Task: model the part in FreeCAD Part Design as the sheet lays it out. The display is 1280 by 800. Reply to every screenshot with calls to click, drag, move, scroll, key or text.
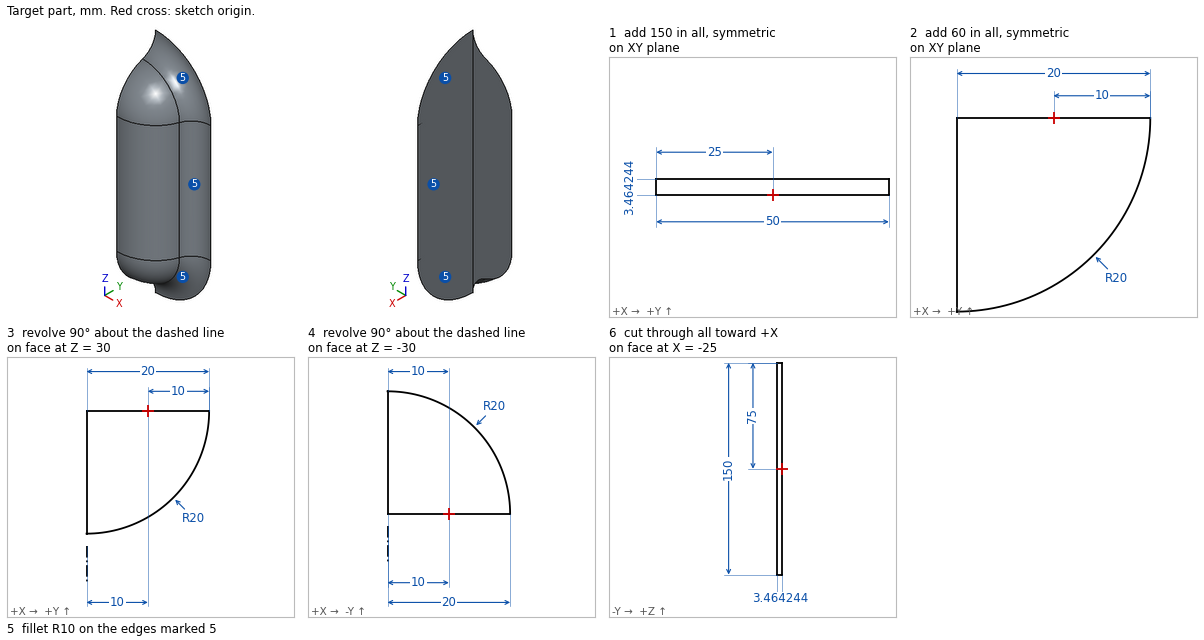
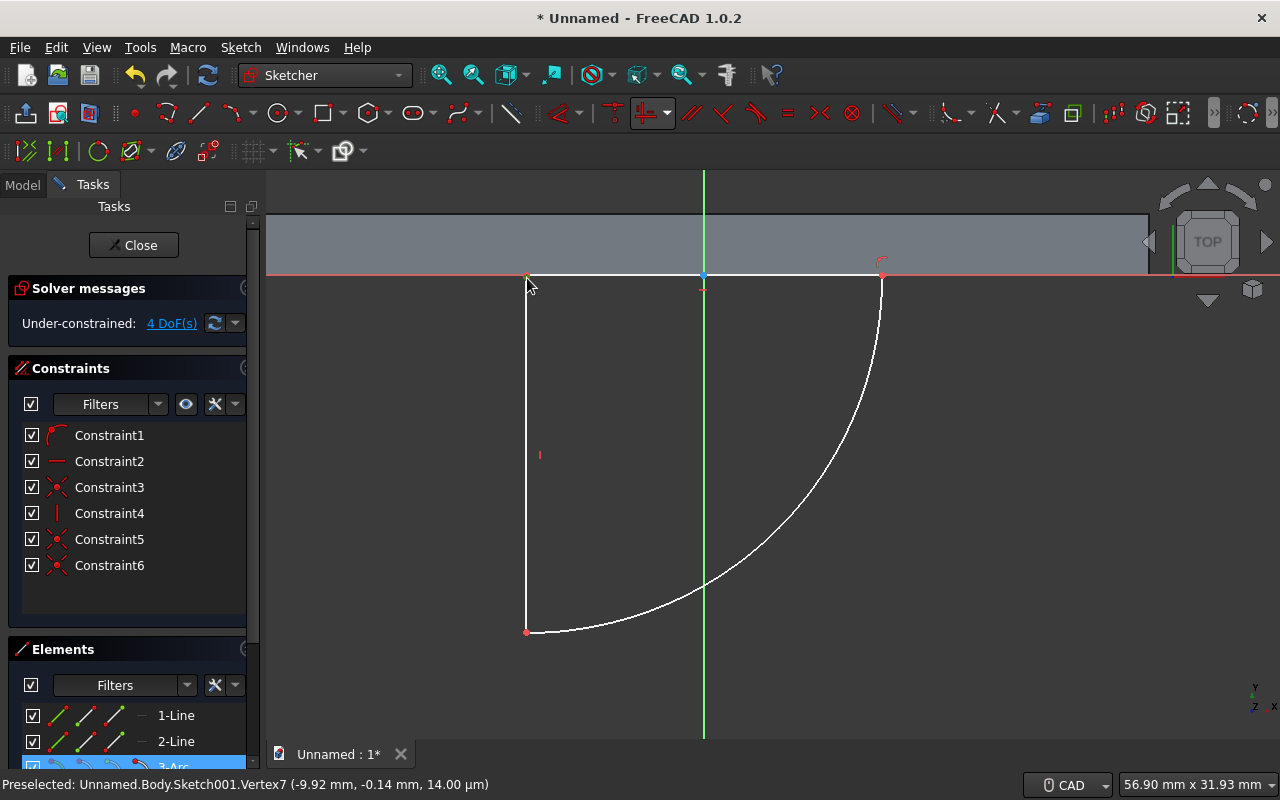
click(353, 275)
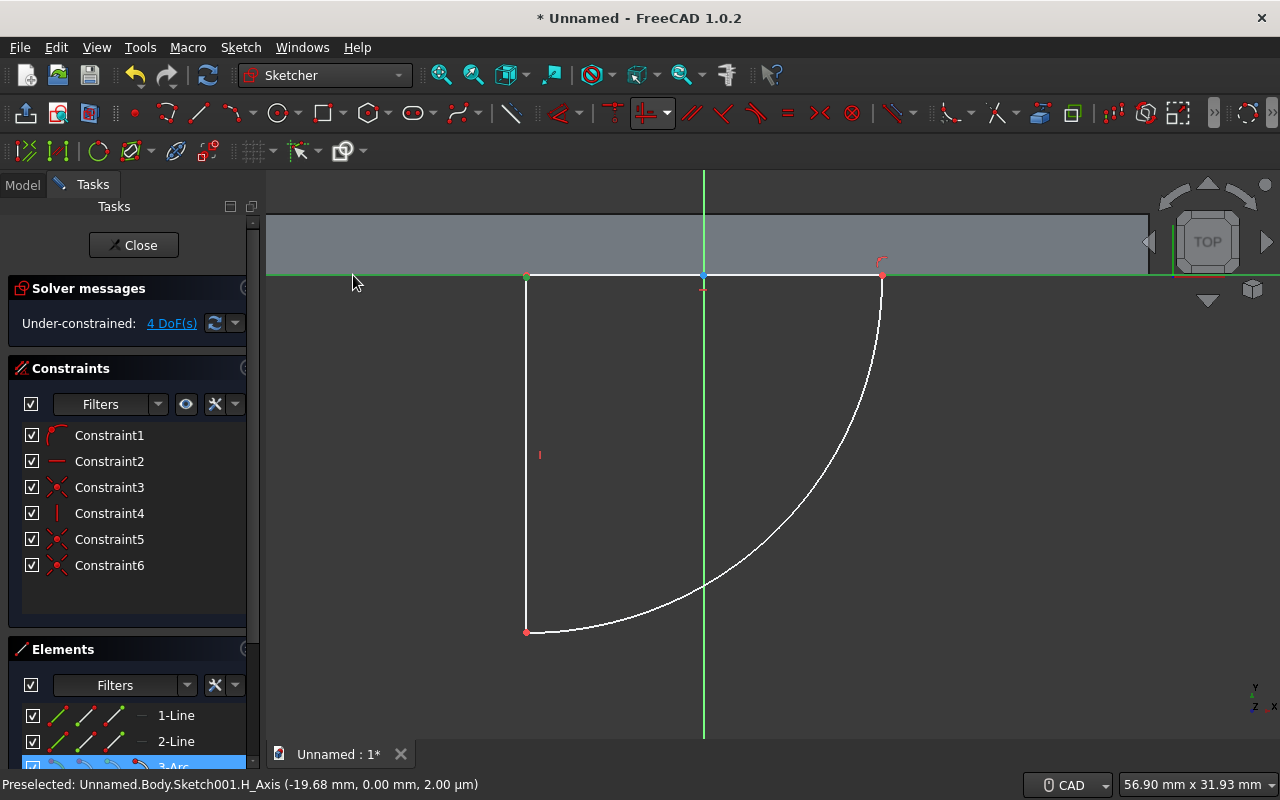
click(614, 114)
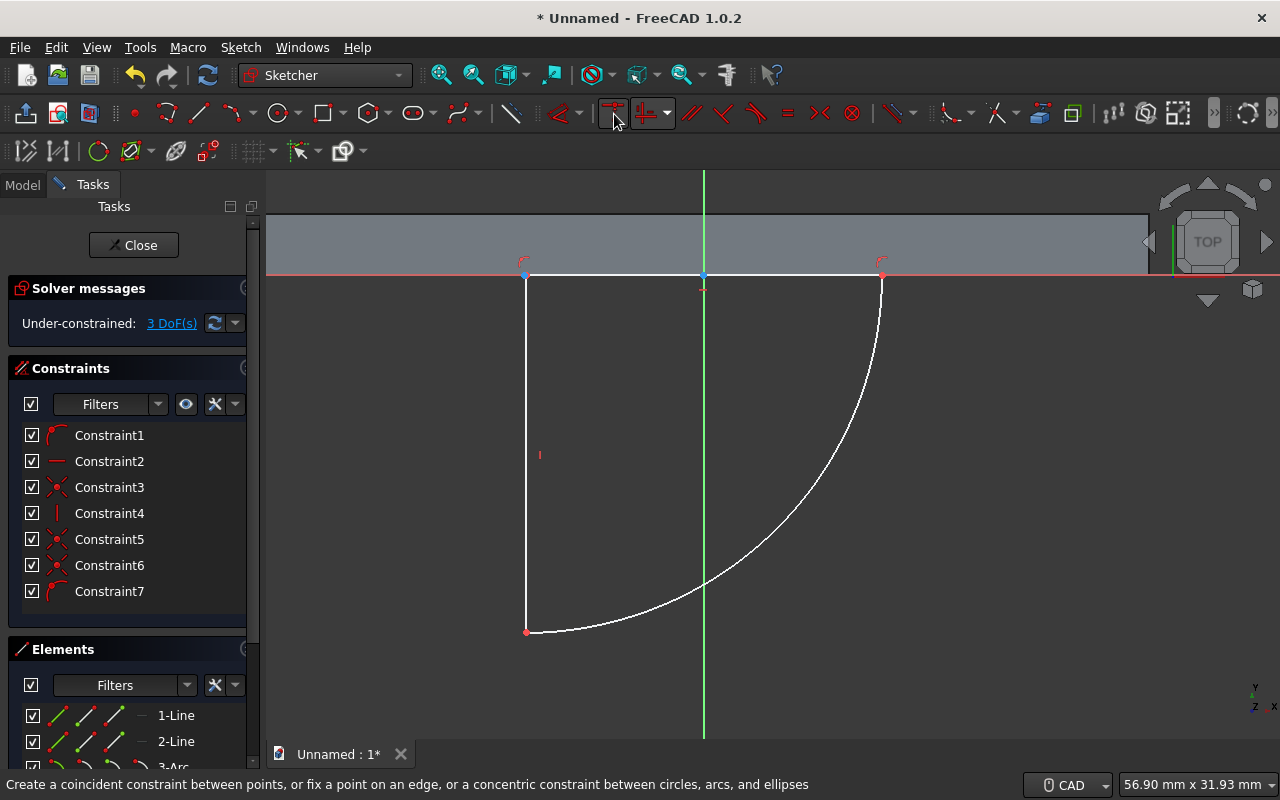
click(558, 114)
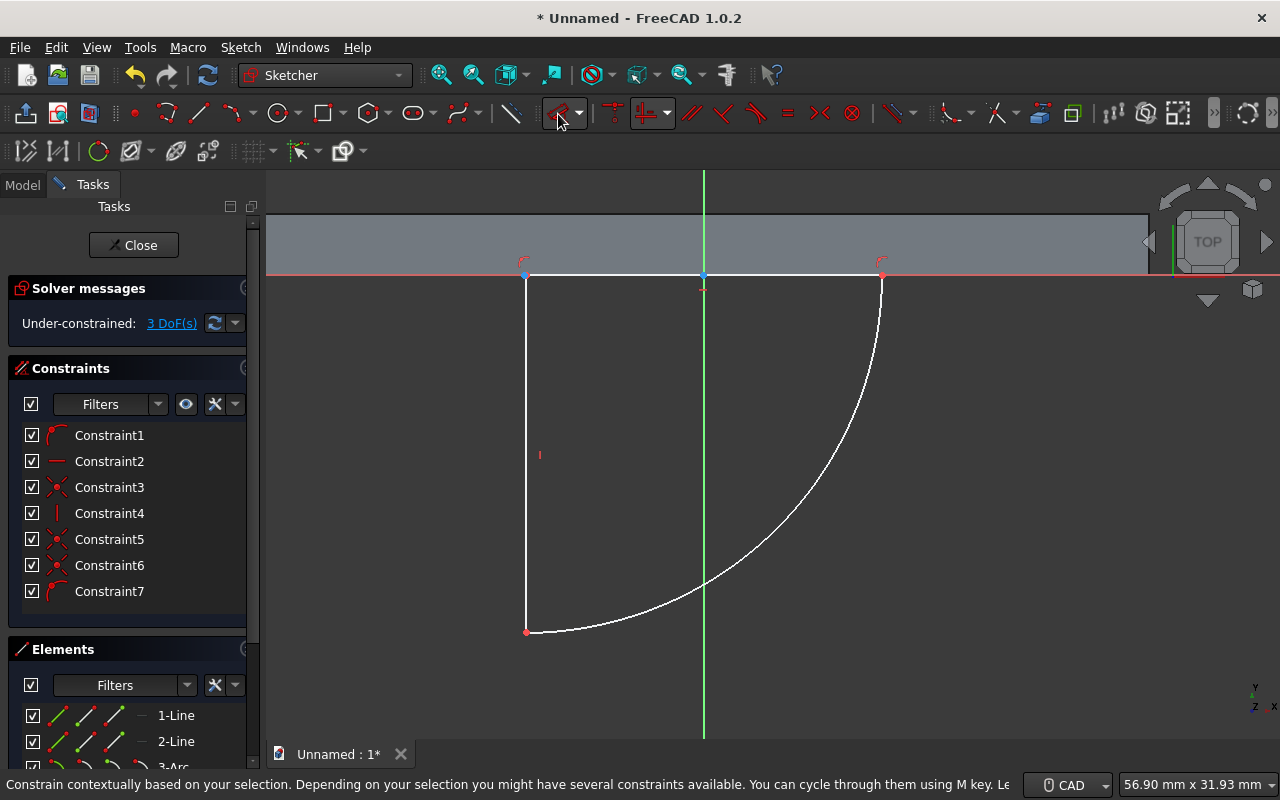
click(688, 594)
click(514, 665)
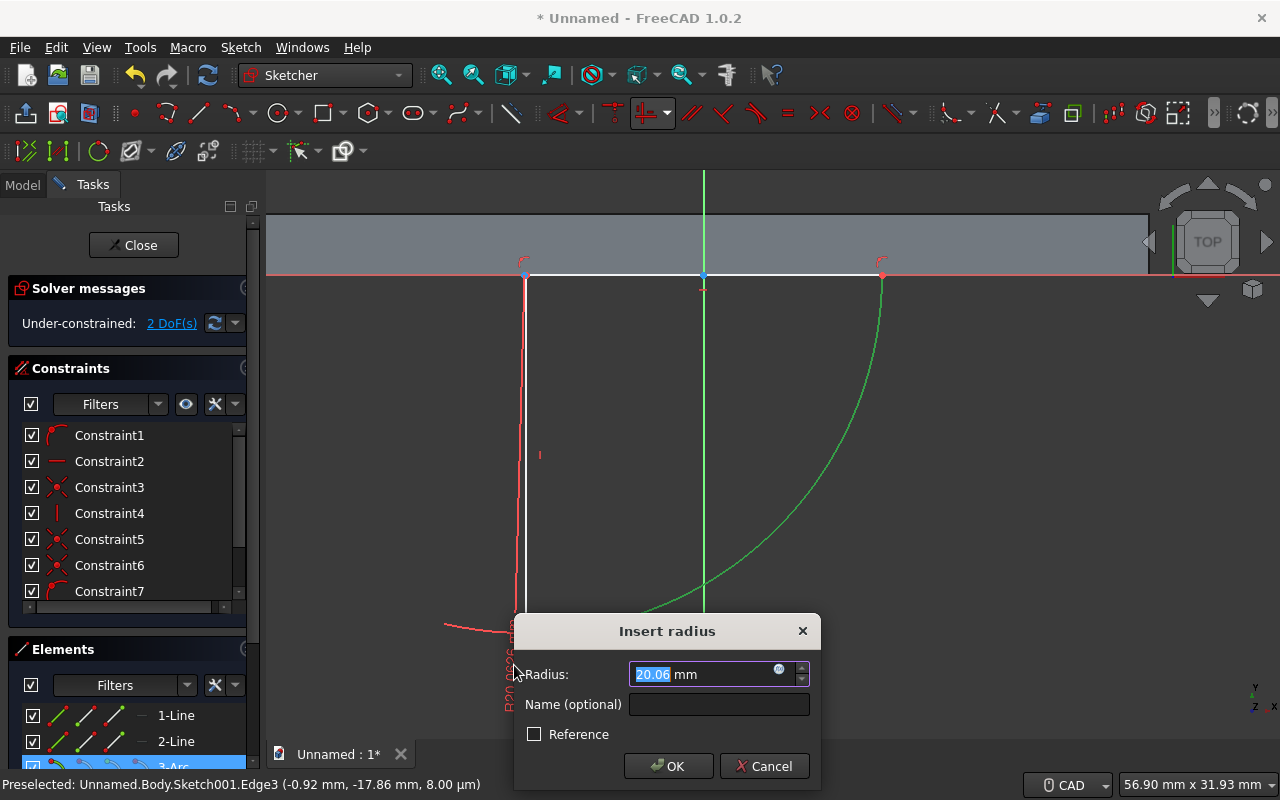
text(20)
key(Return)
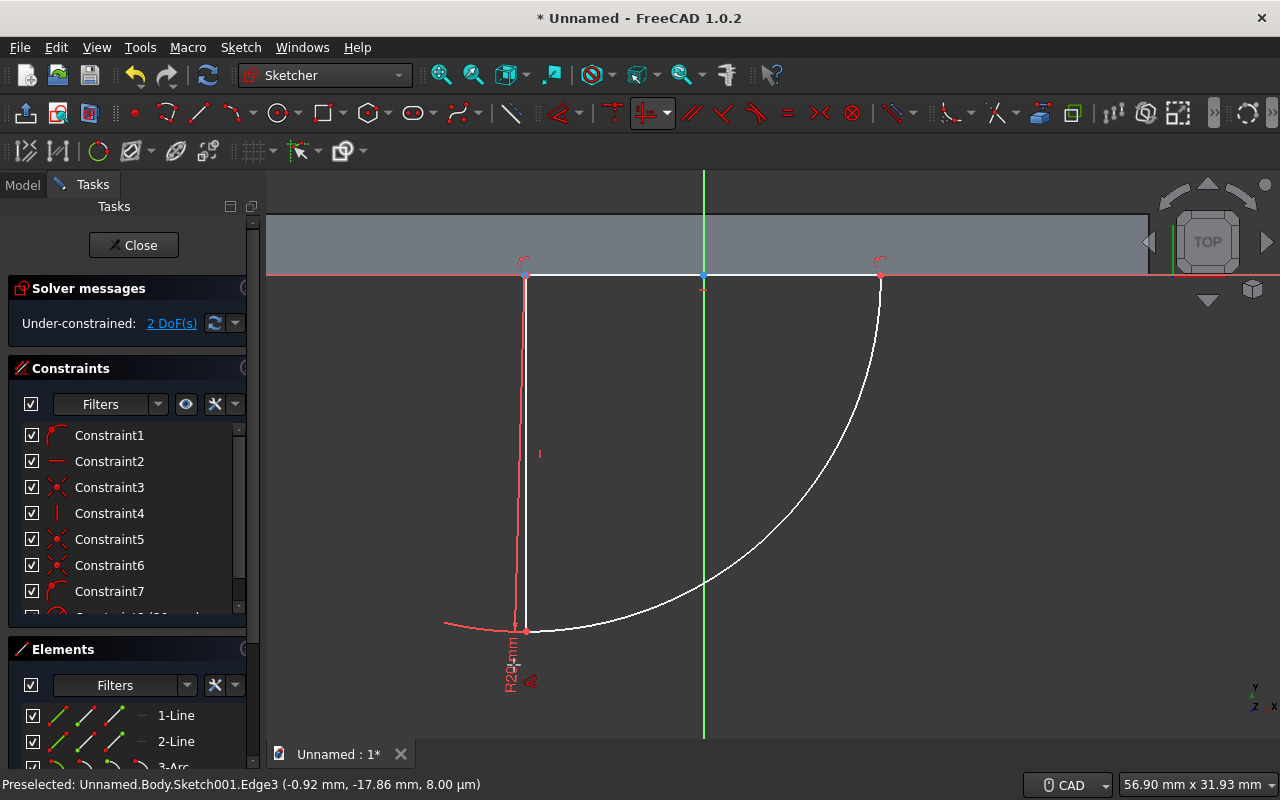
click(774, 275)
click(622, 241)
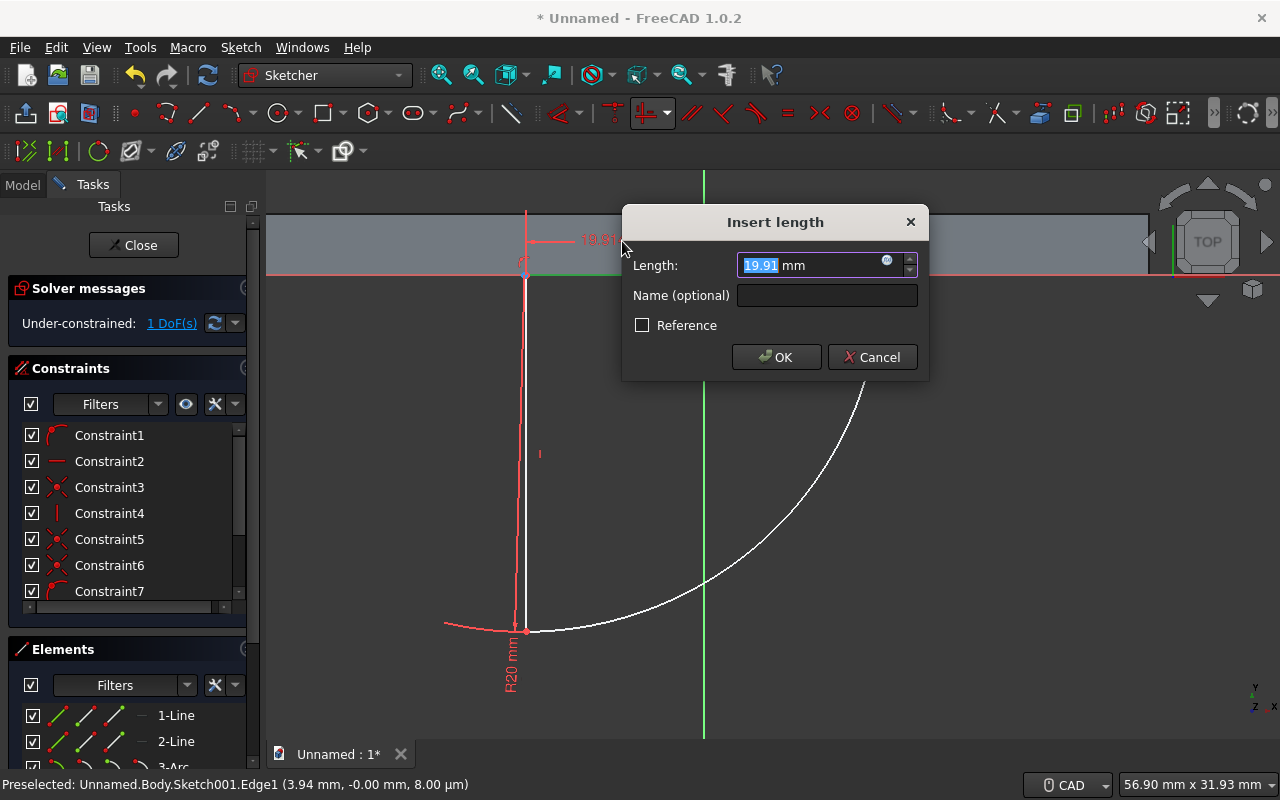
text(20)
key(Return)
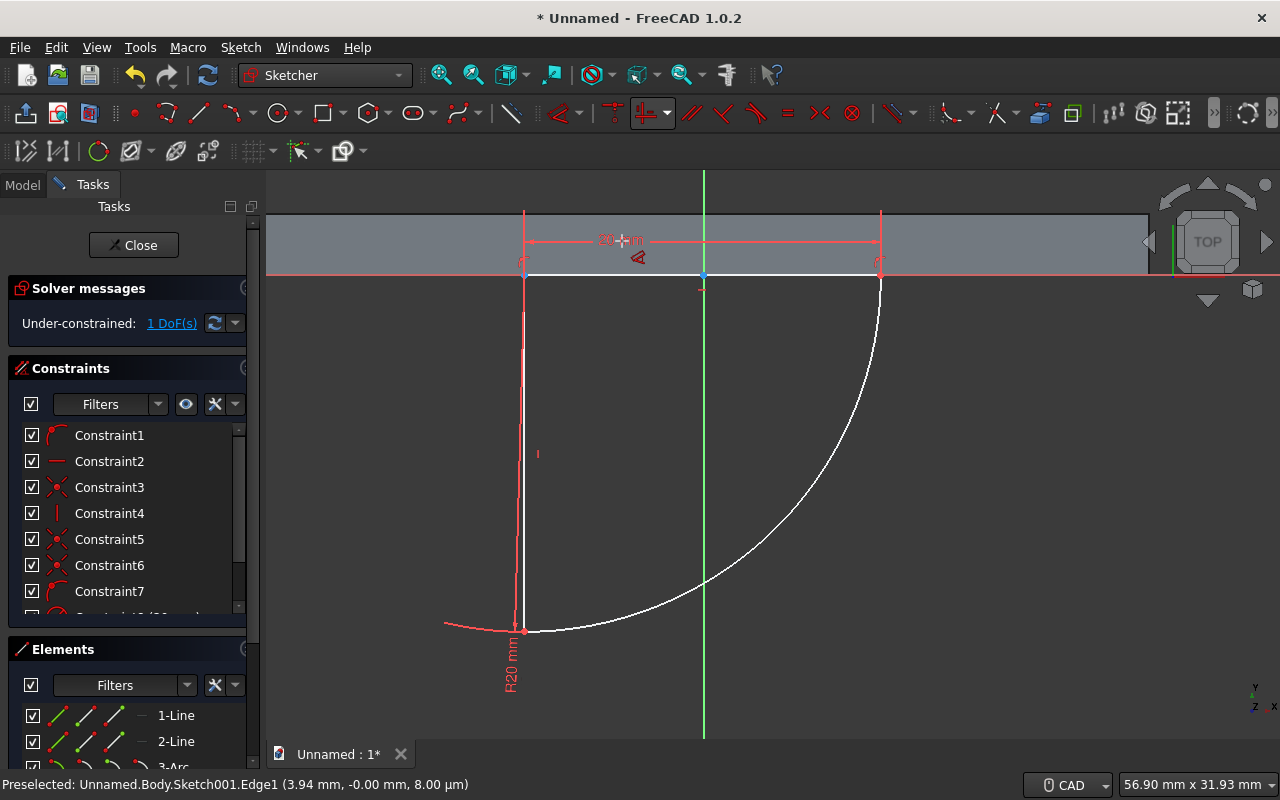
click(881, 275)
click(792, 241)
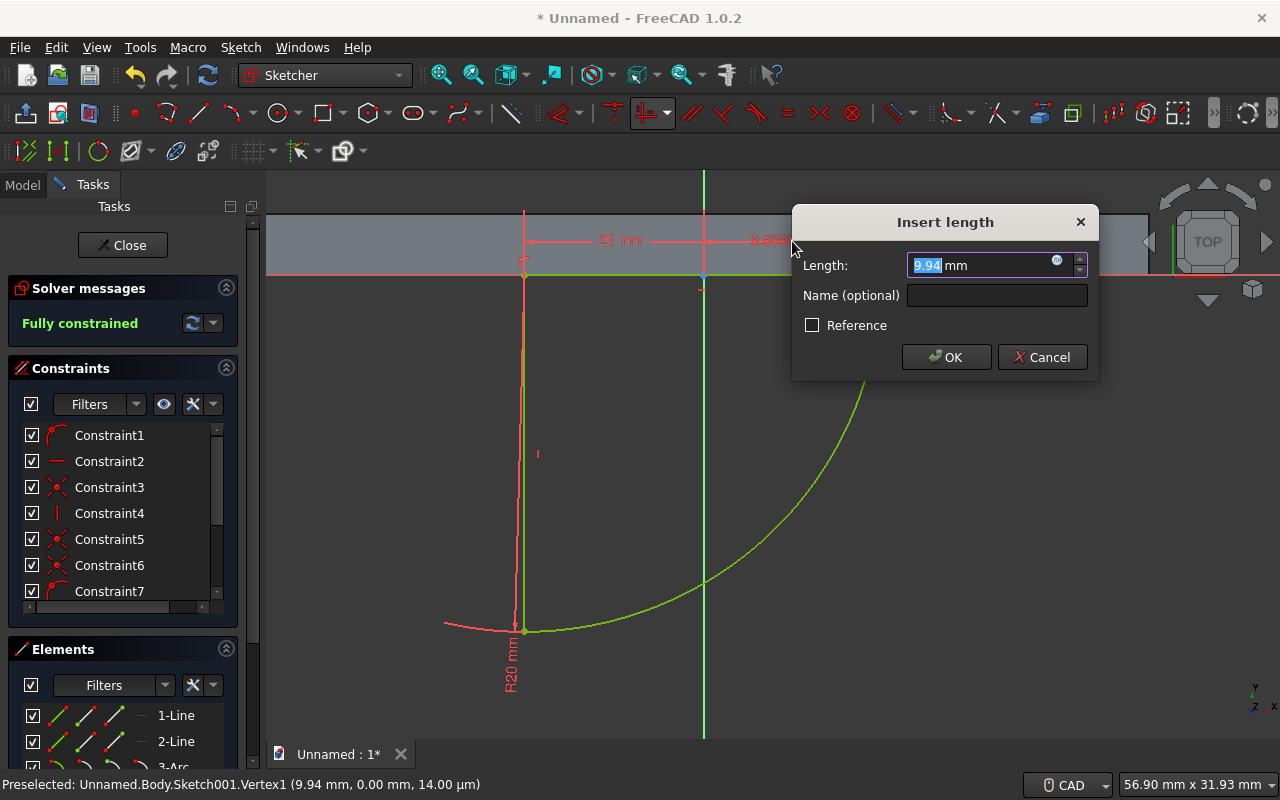
text(10)
key(Return)
key(Escape)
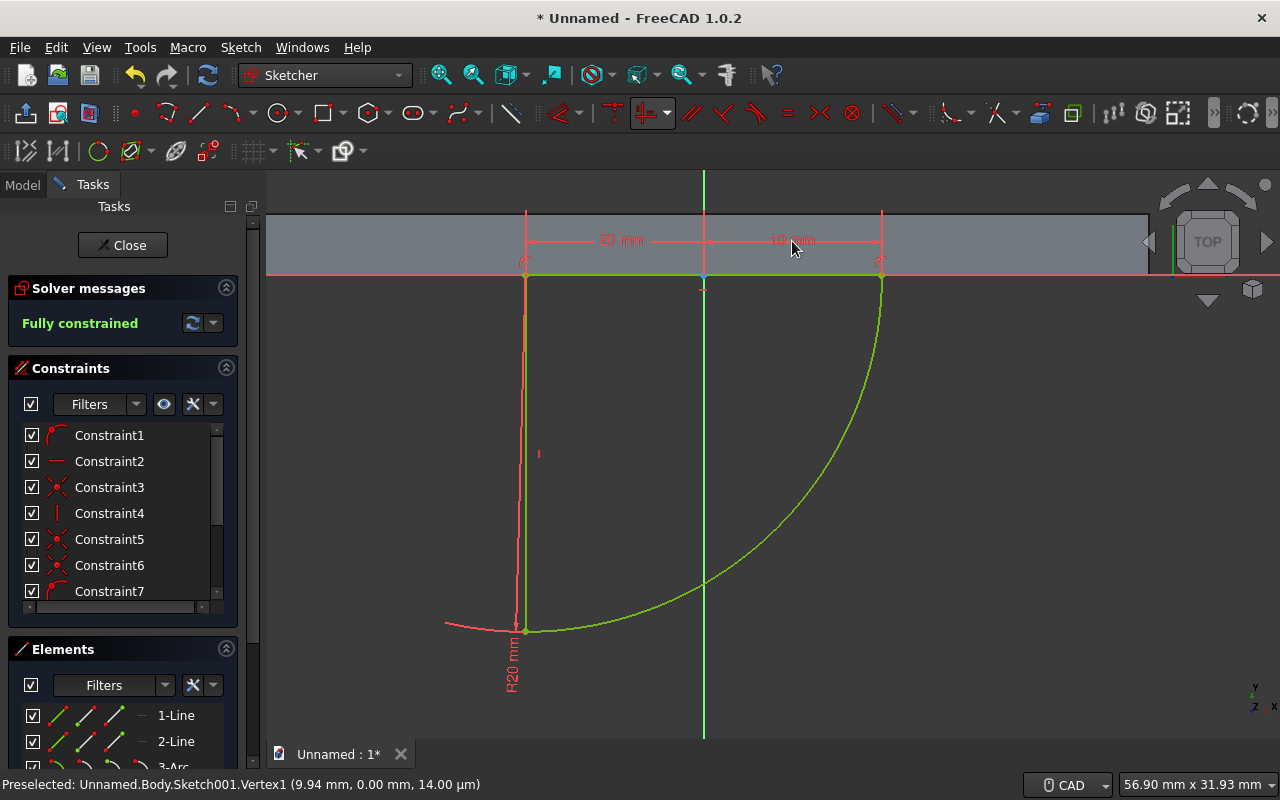
click(123, 245)